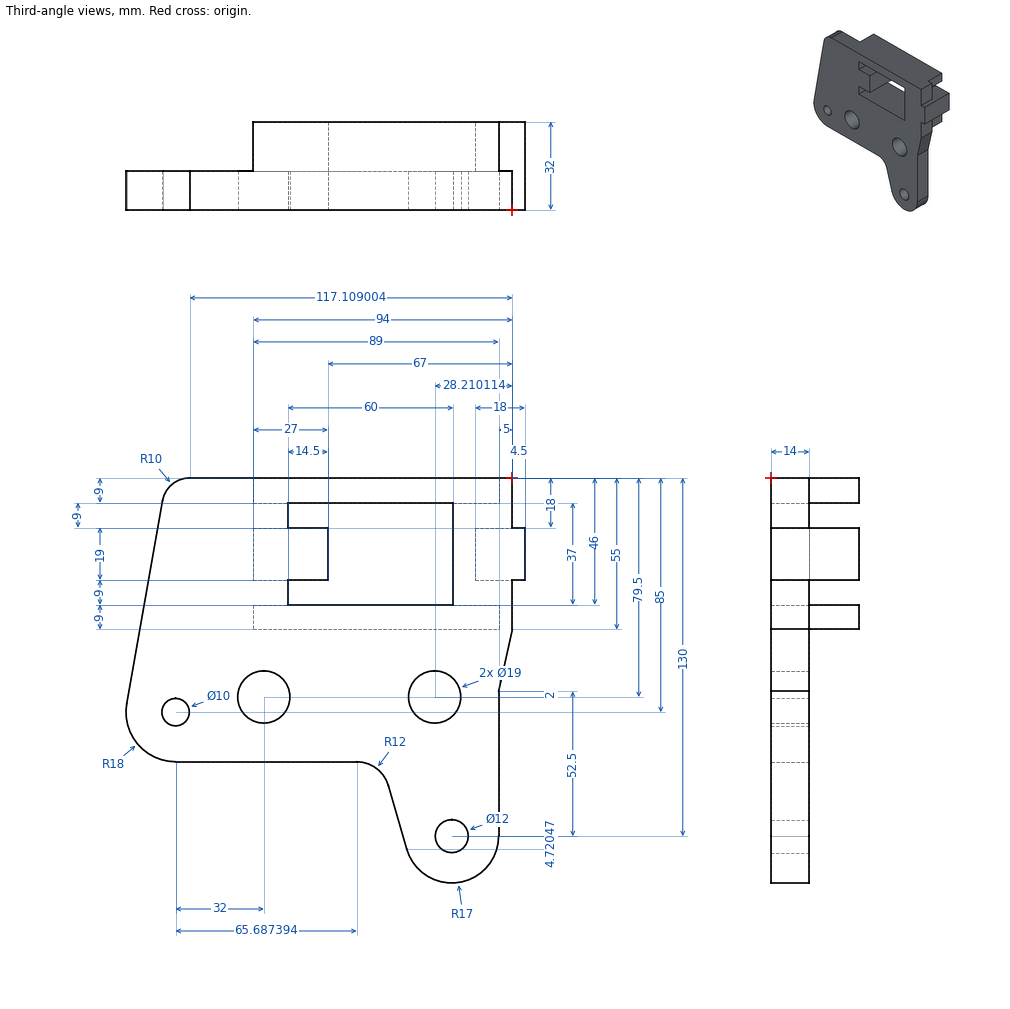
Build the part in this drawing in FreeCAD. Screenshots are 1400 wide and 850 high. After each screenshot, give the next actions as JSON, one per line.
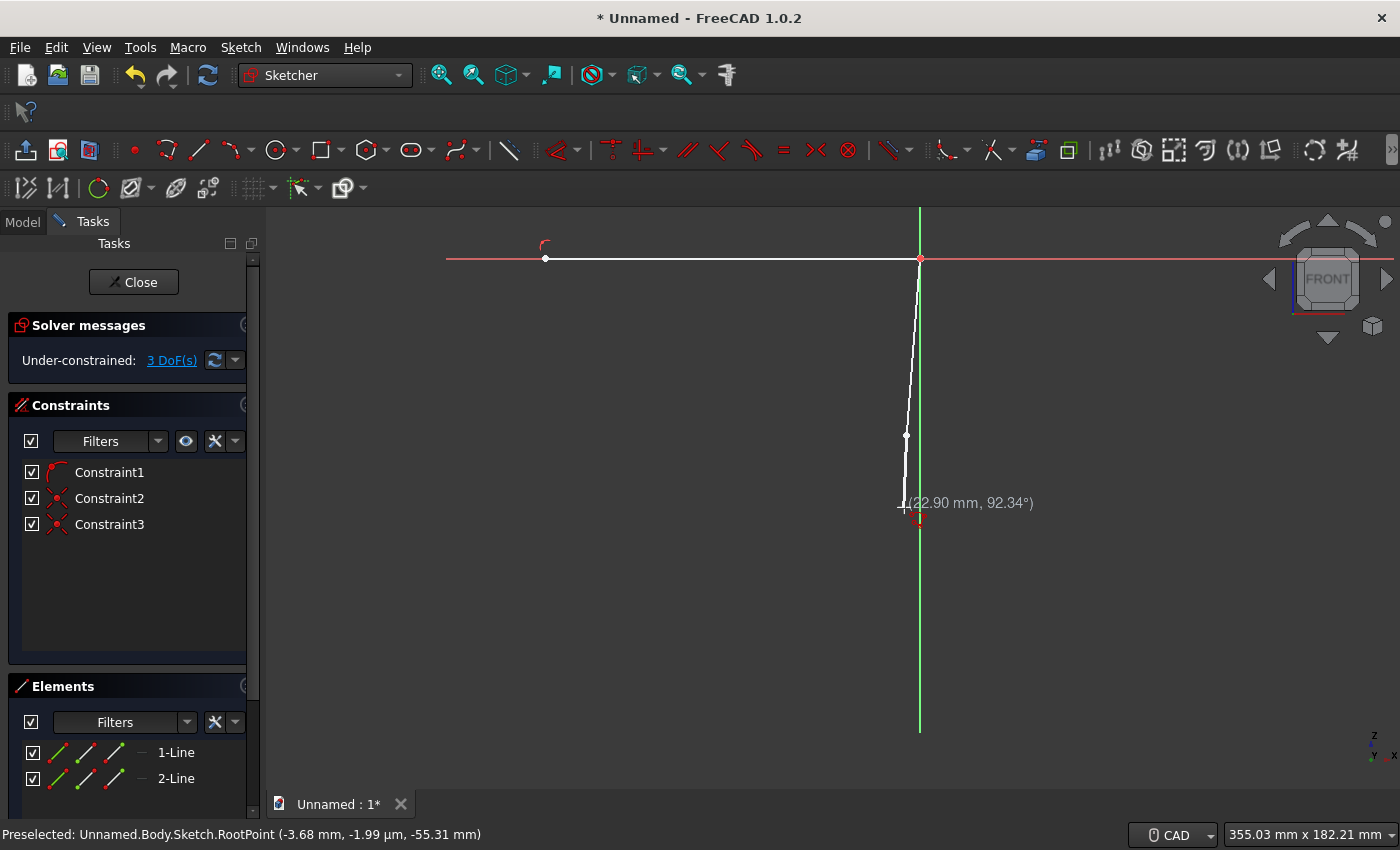
{"action": "left_click", "coordinate": [904, 506]}
{"action": "left_click", "coordinate": [904, 674]}
{"action": "right_click", "coordinate": [904, 674]}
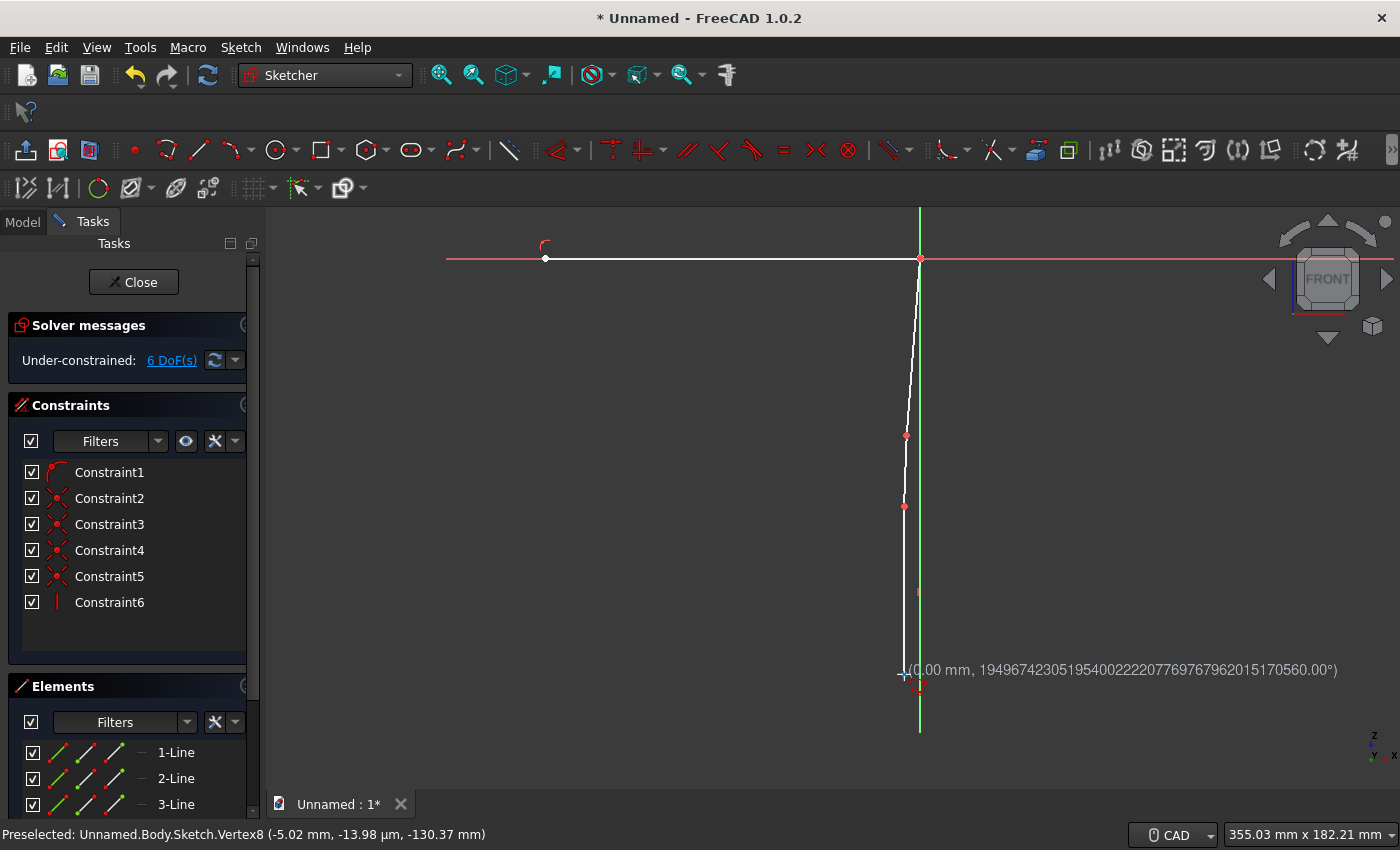
{"action": "left_click", "coordinate": [200, 150]}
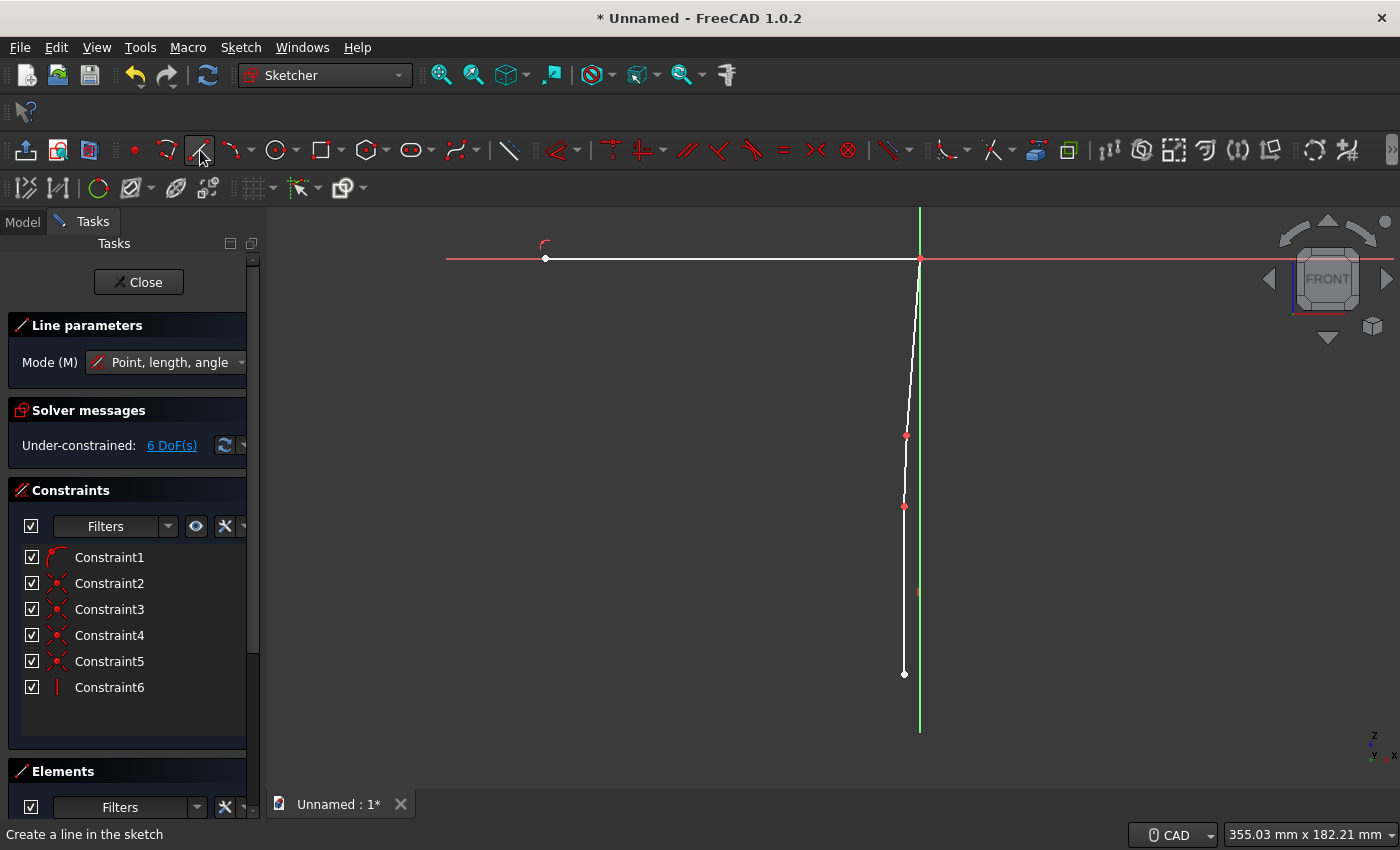
{"action": "left_click", "coordinate": [798, 689]}
{"action": "left_click", "coordinate": [776, 615]}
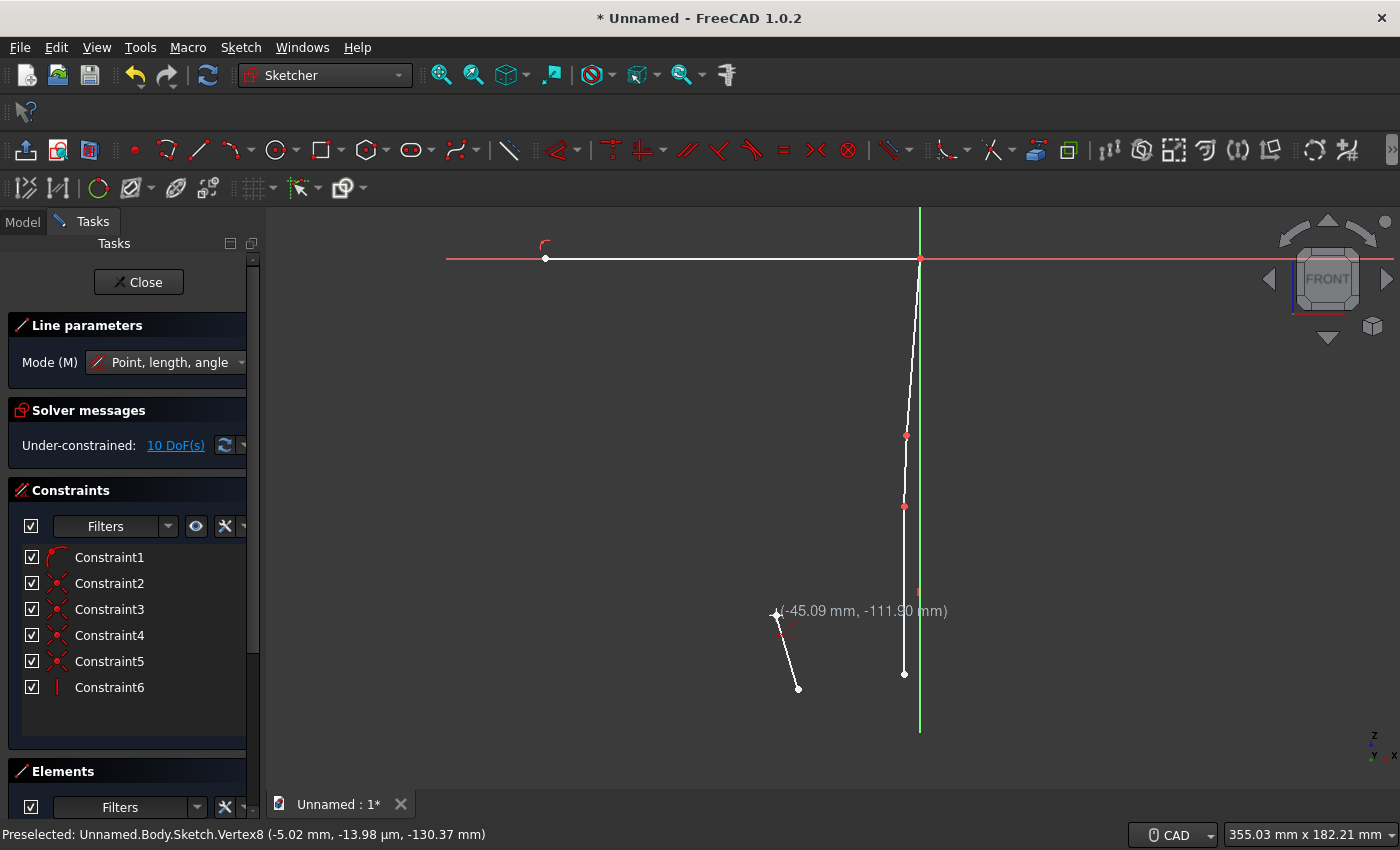
{"action": "left_click", "coordinate": [739, 588]}
{"action": "left_click", "coordinate": [530, 588]}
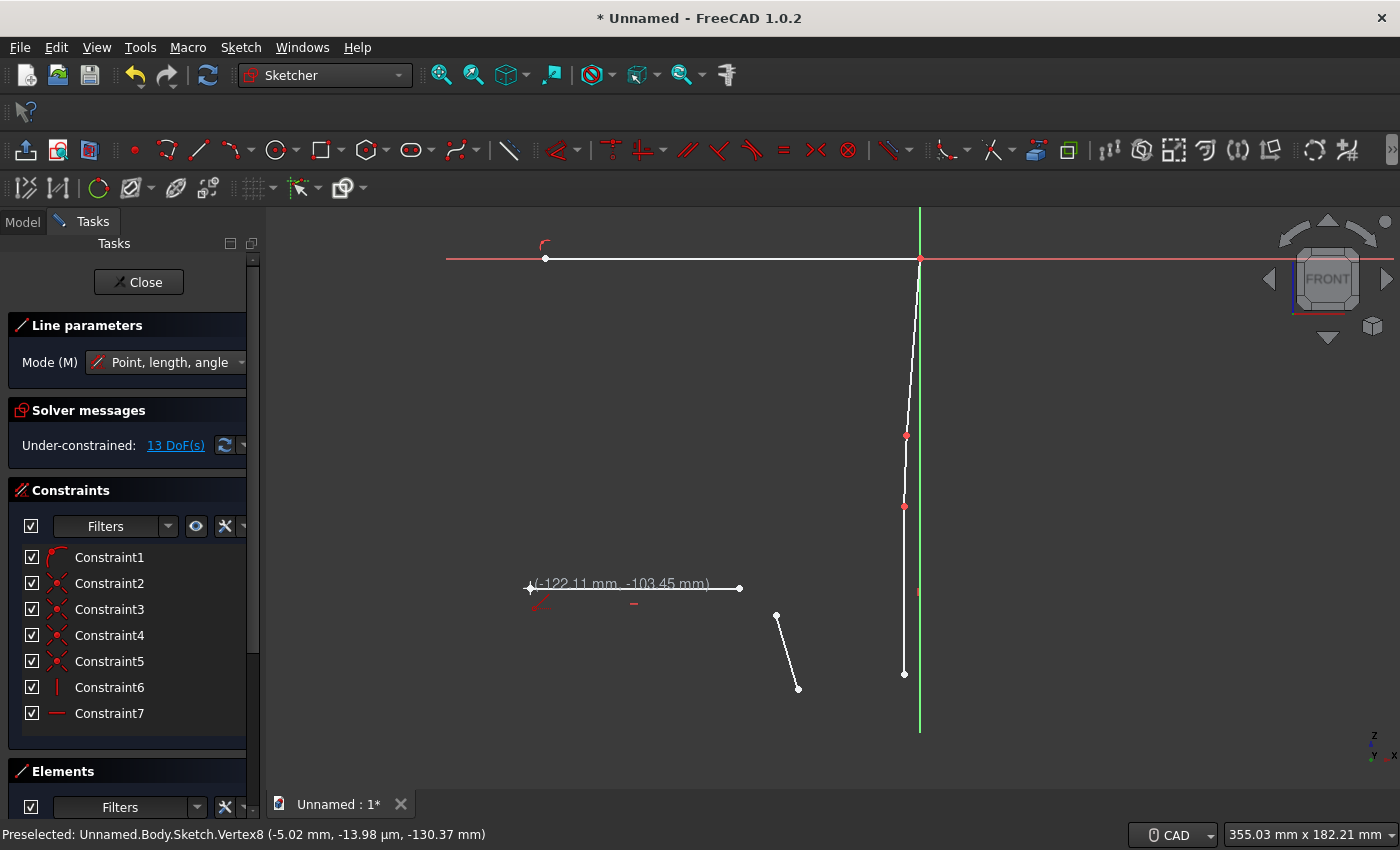
{"action": "left_click", "coordinate": [473, 520]}
{"action": "left_click", "coordinate": [515, 285]}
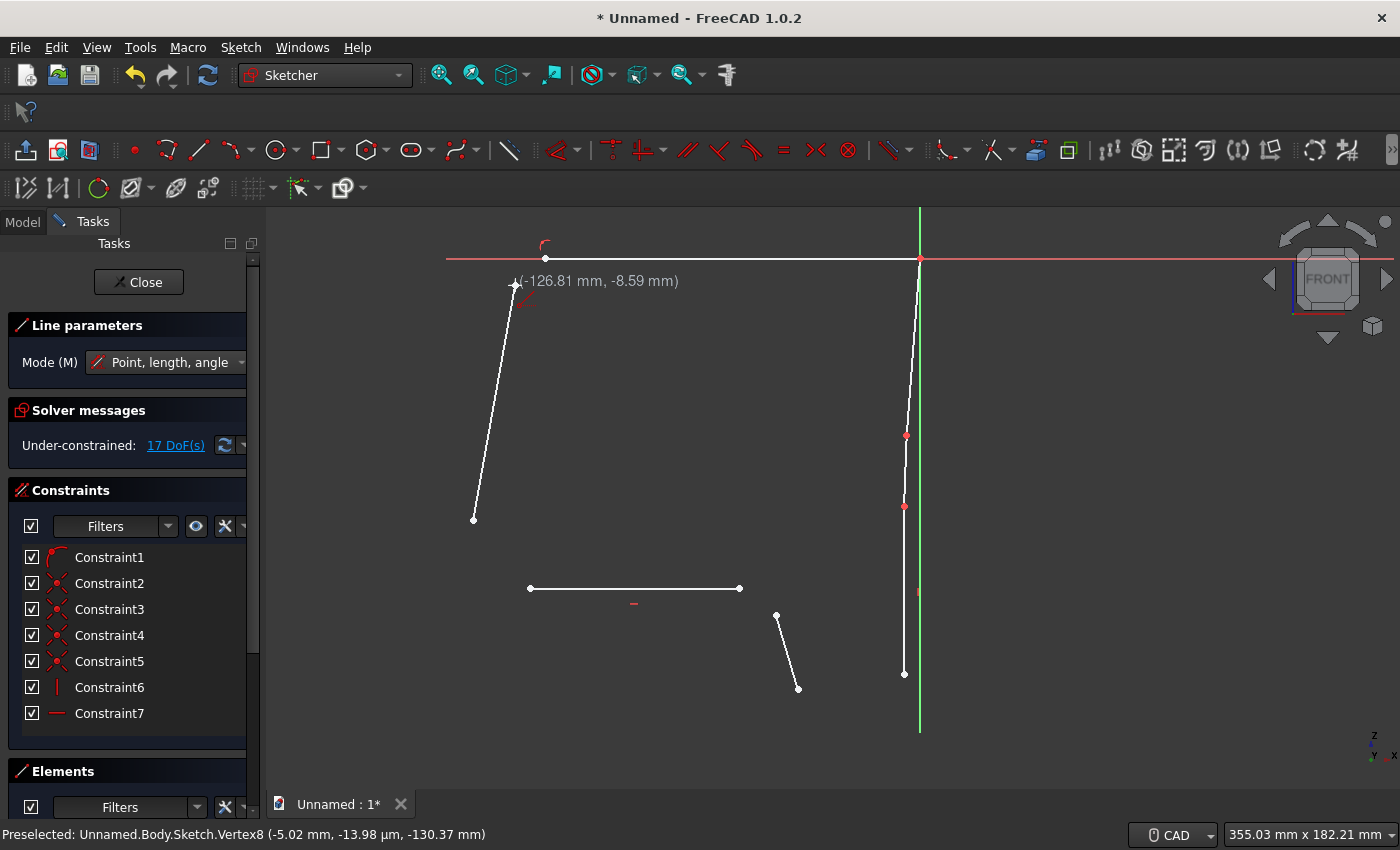
{"action": "left_click", "coordinate": [232, 150]}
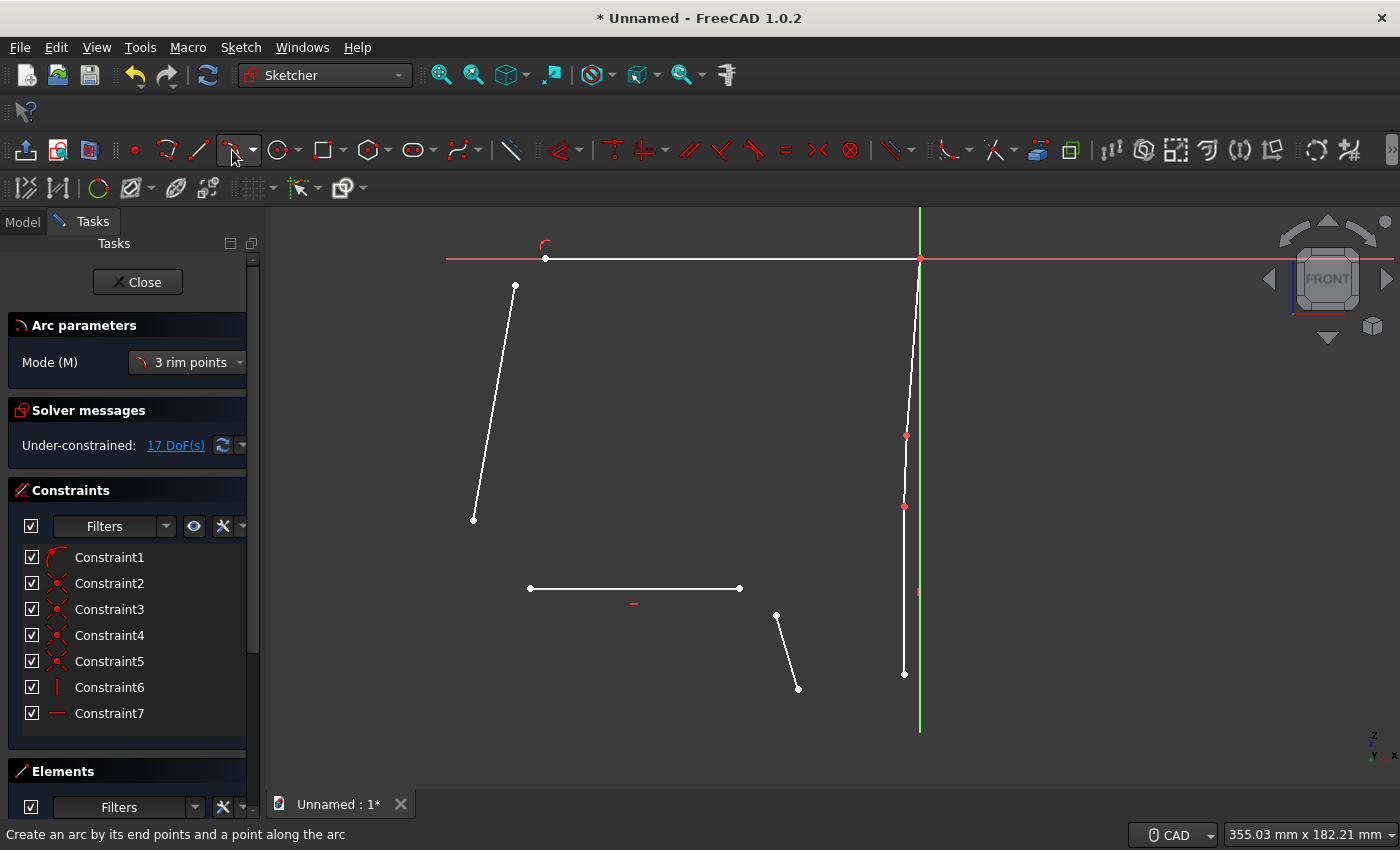
{"action": "left_click", "coordinate": [904, 675]}
{"action": "left_click", "coordinate": [798, 690]}
{"action": "left_click", "coordinate": [857, 728]}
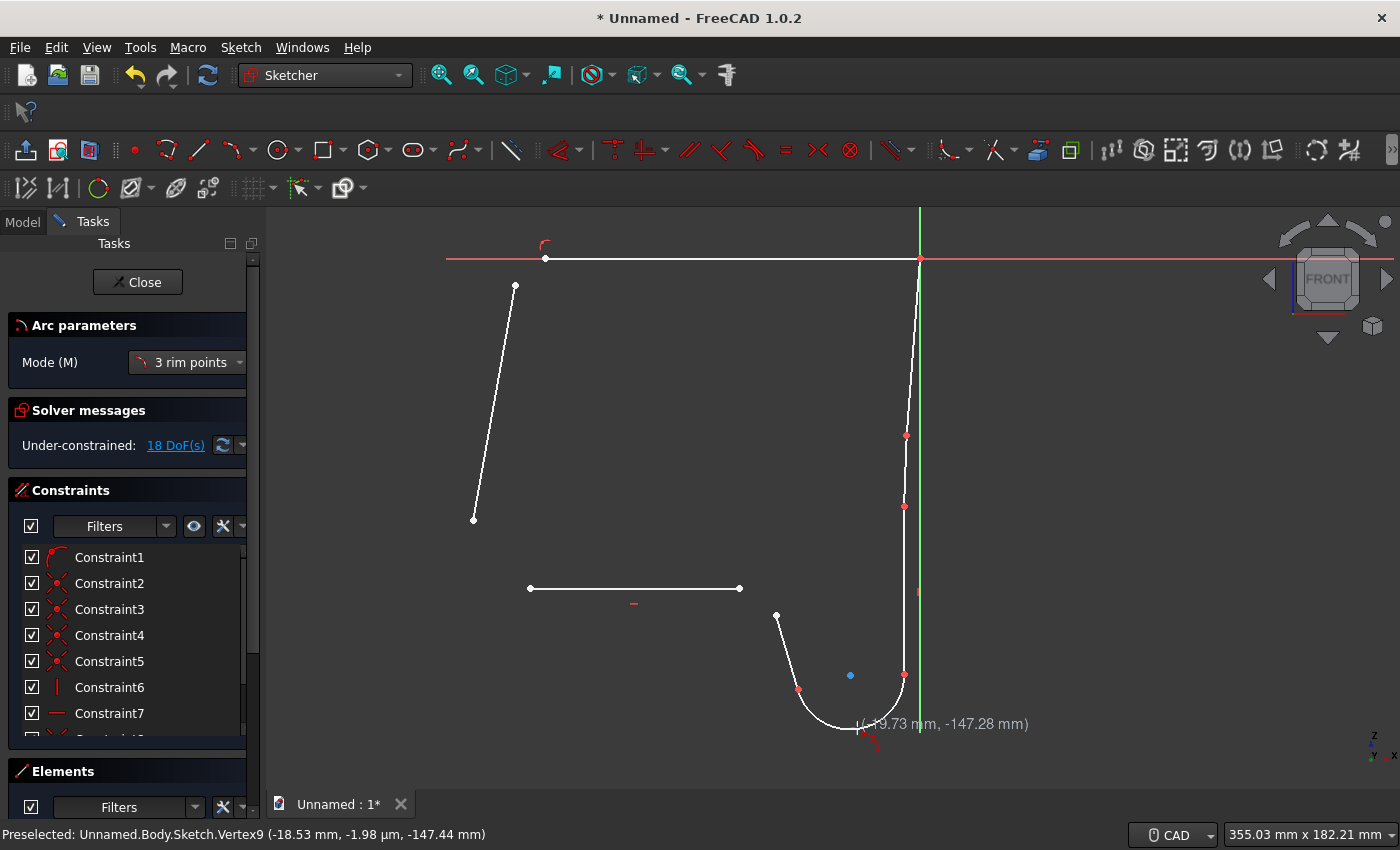
{"action": "left_click", "coordinate": [776, 616]}
{"action": "left_click", "coordinate": [739, 589]}